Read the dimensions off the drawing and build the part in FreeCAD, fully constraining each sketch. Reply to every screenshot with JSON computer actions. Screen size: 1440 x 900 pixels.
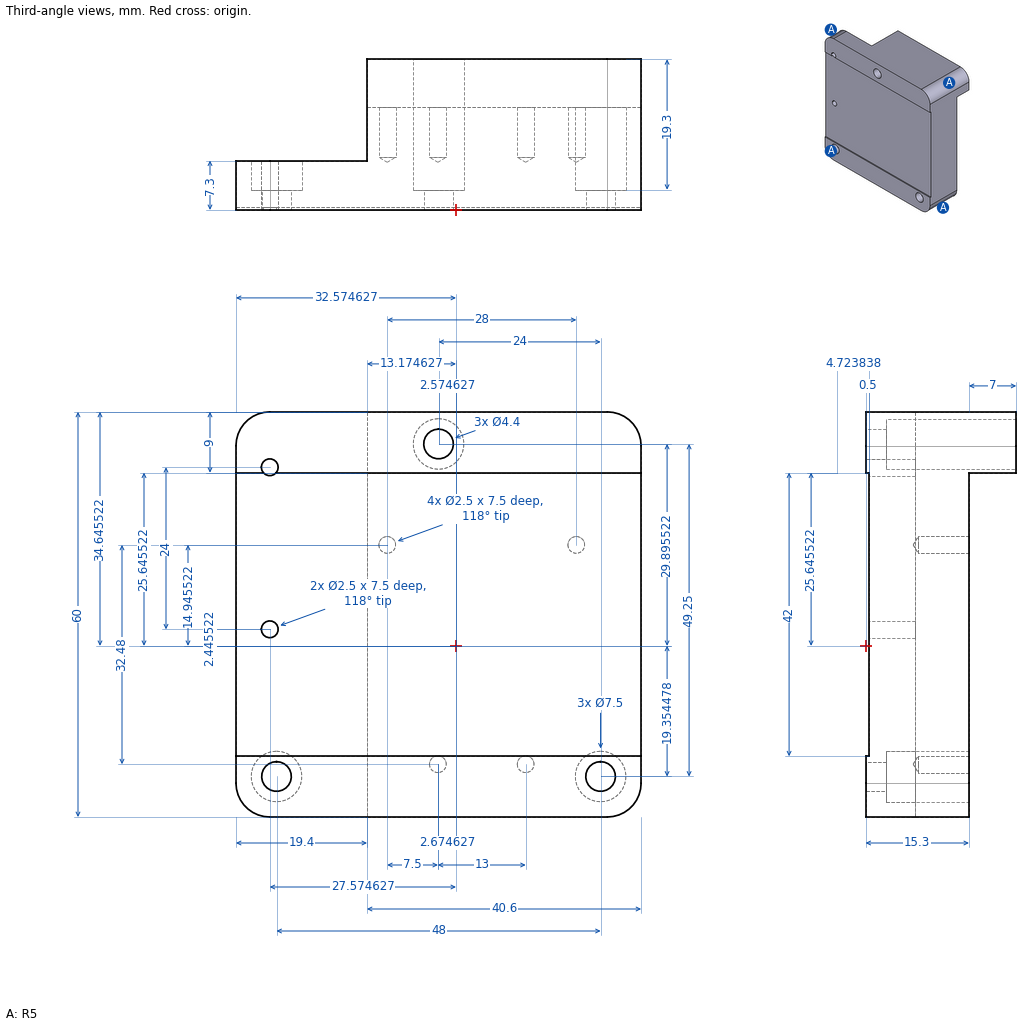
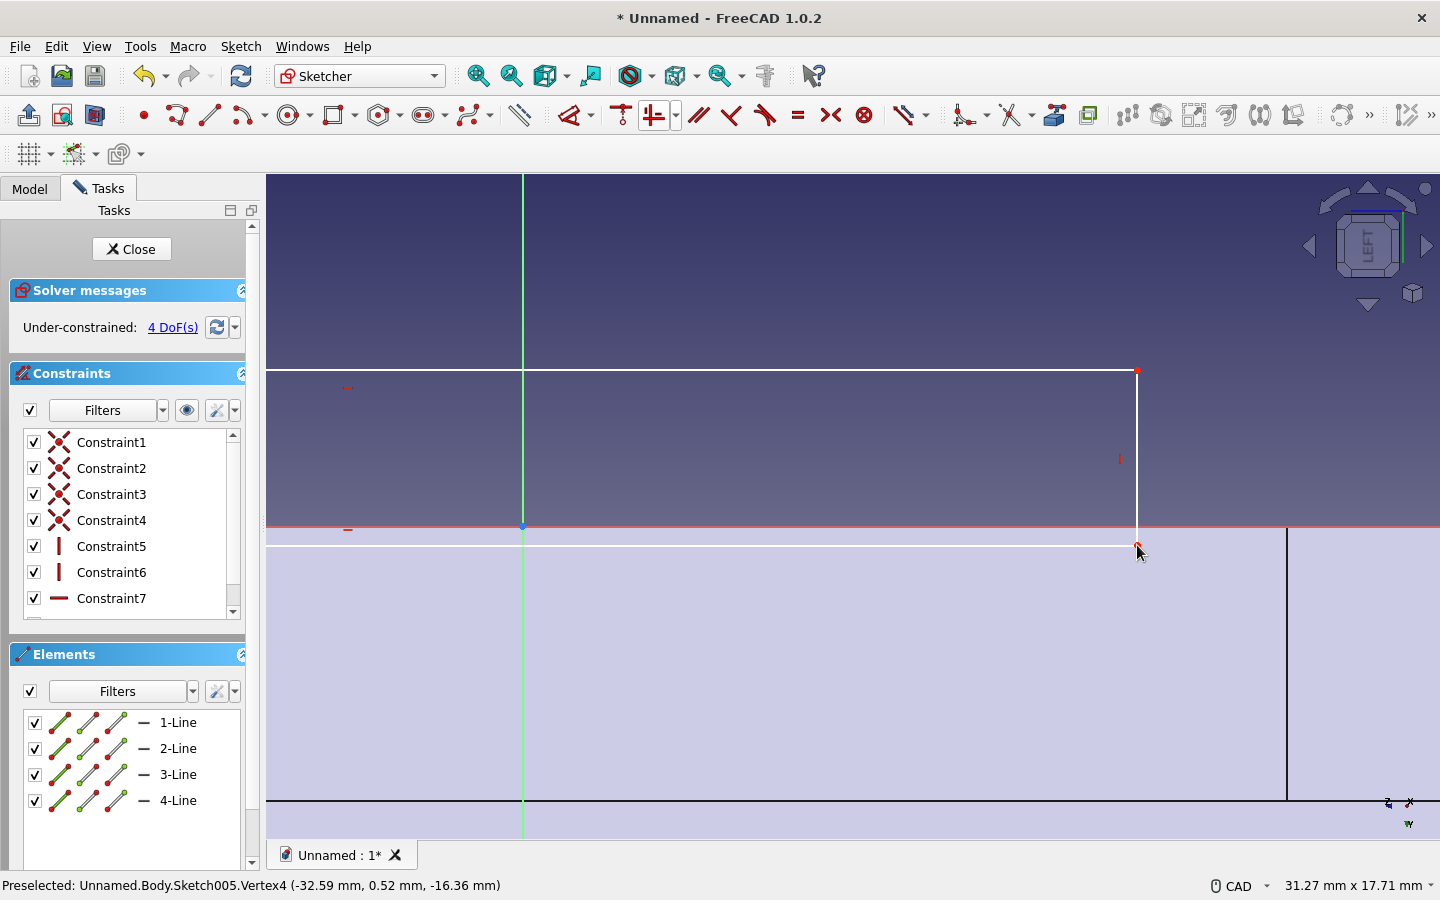
{"action": "key", "text": "d"}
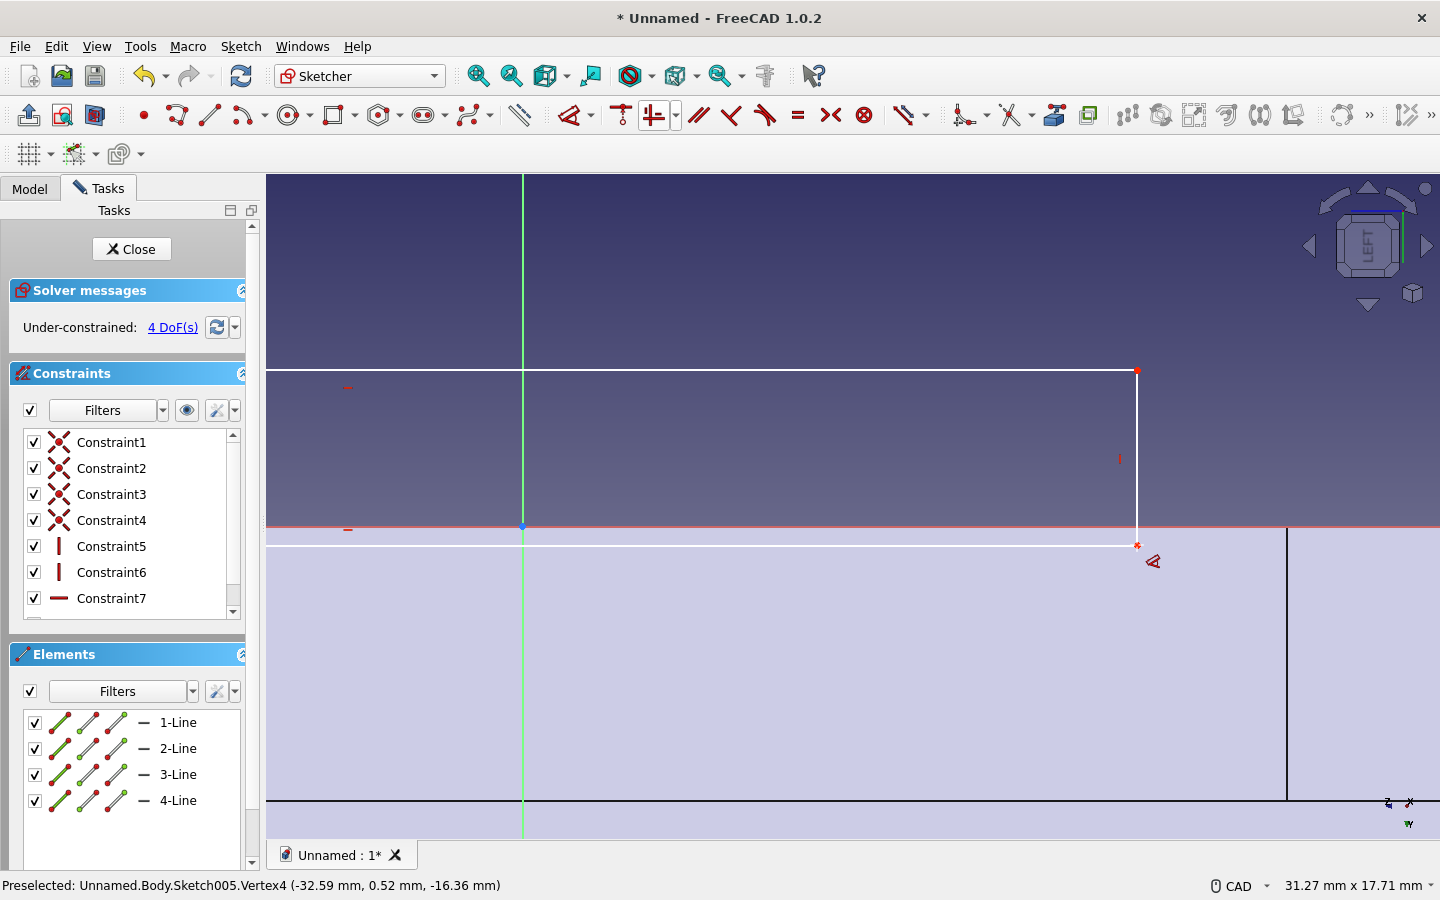
{"action": "left_click", "coordinate": [664, 546]}
{"action": "left_click", "coordinate": [715, 580]}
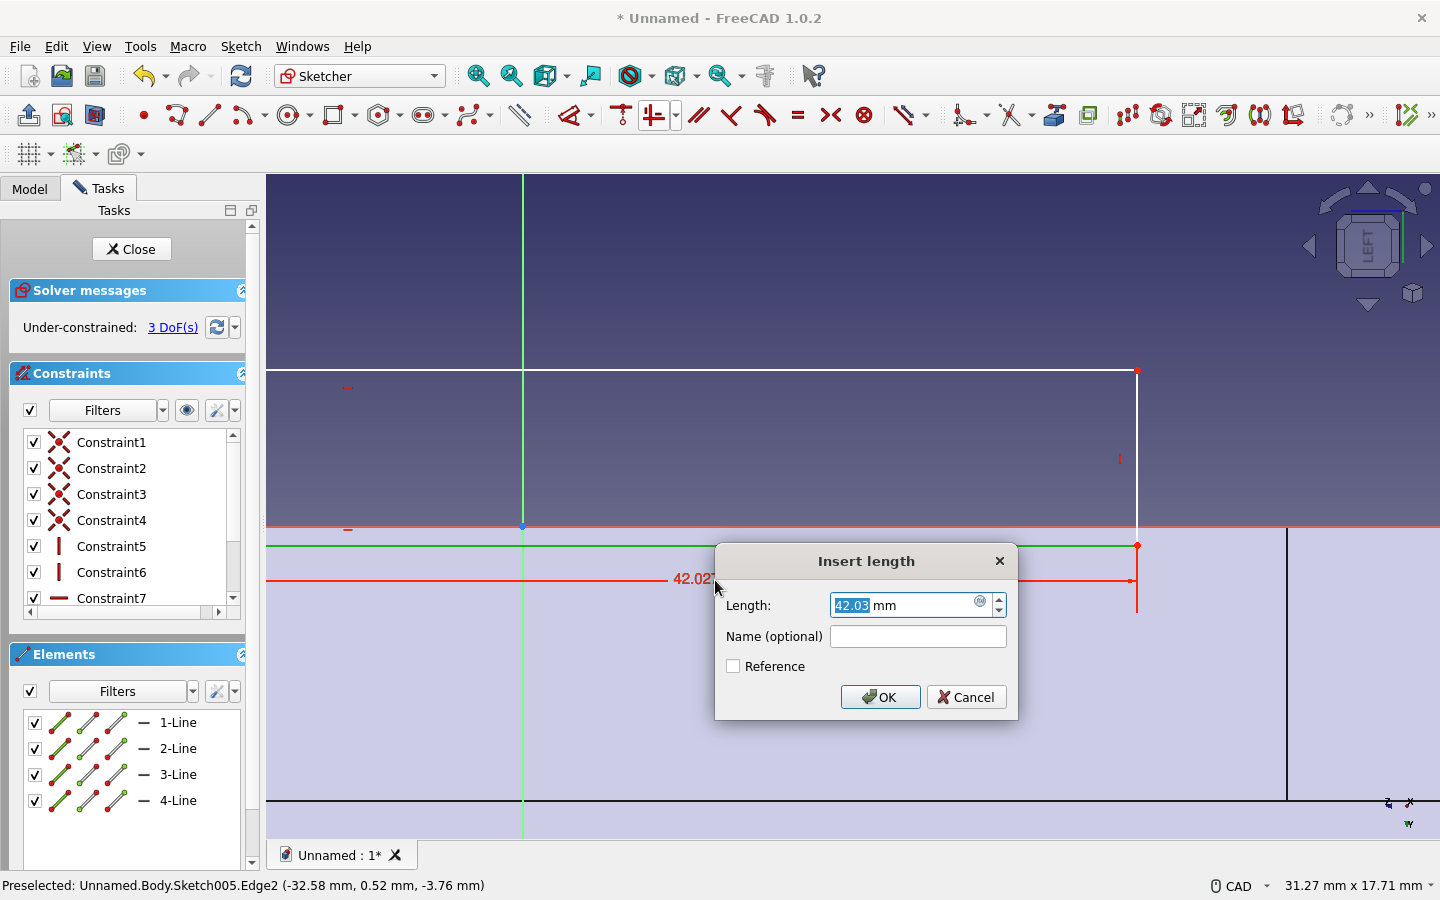
{"action": "type", "text": "42"}
{"action": "key", "text": "Return"}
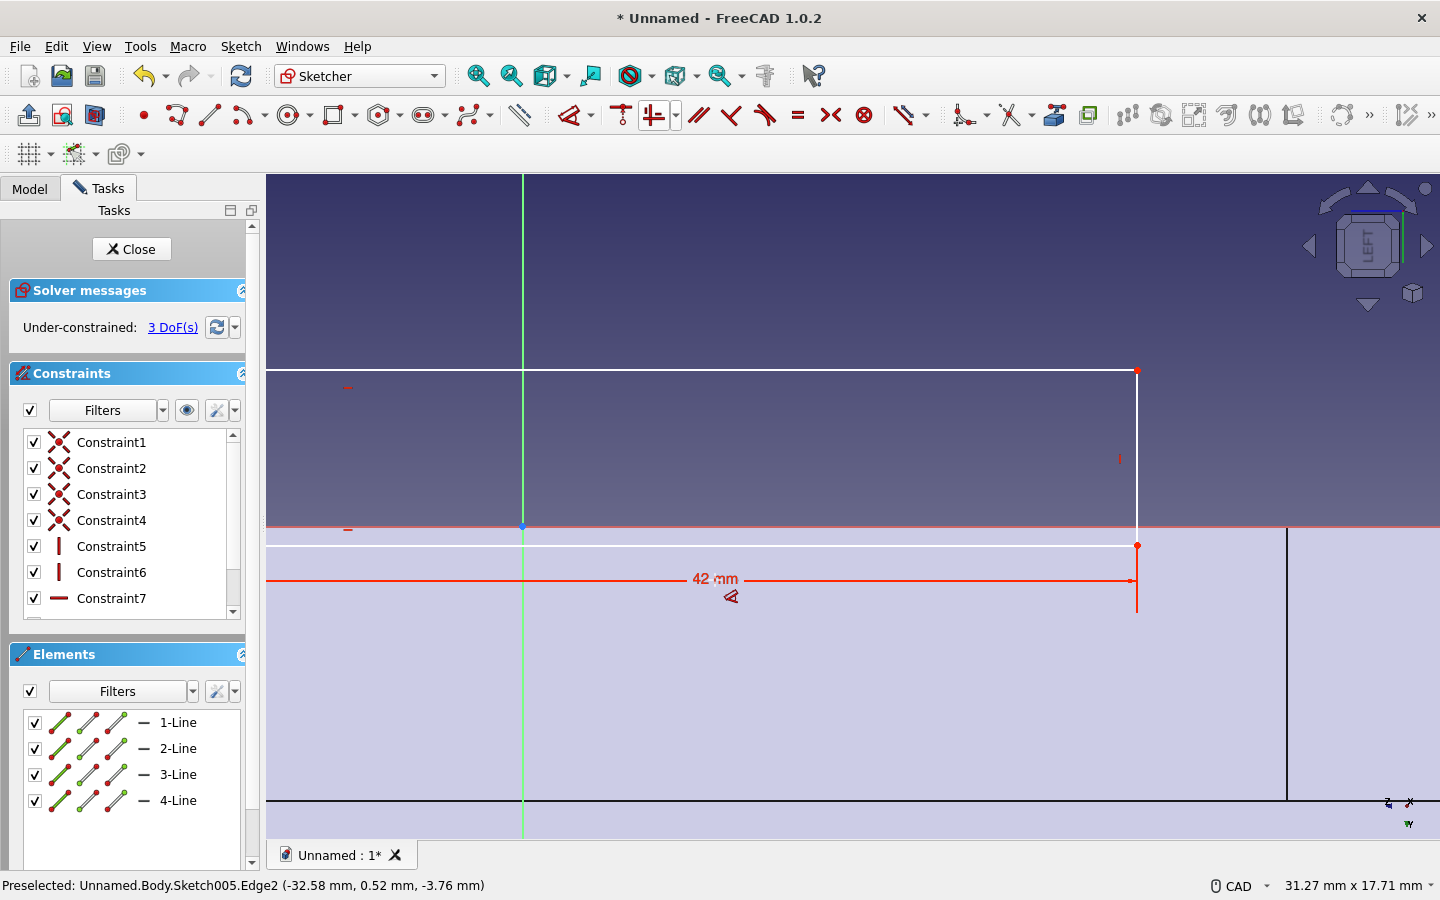
{"action": "scroll", "coordinate": [1140, 547], "scroll_direction": "down", "scroll_amount": 4}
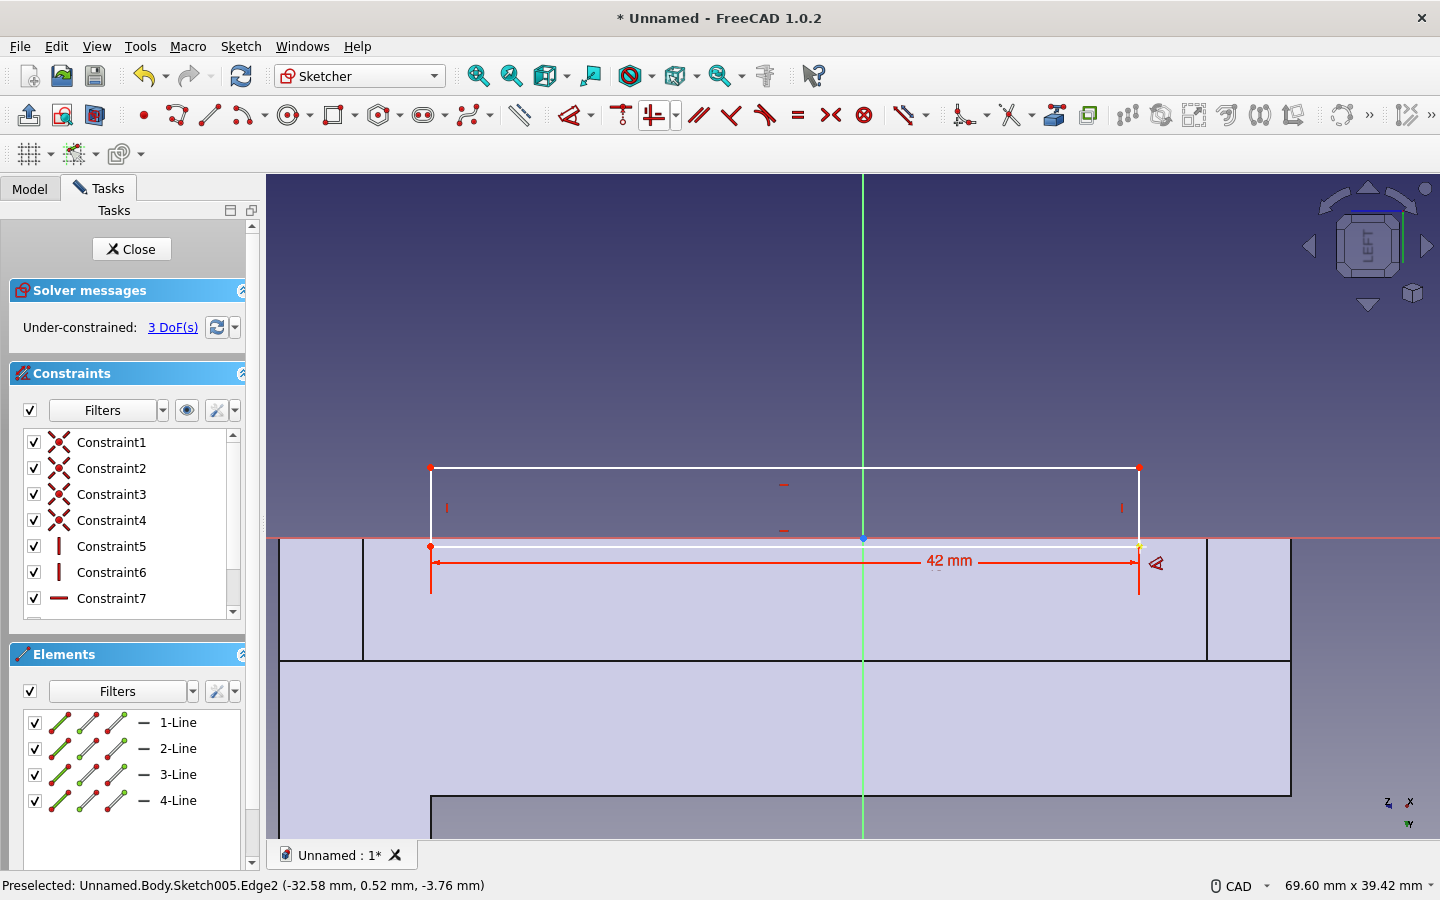
{"action": "scroll", "coordinate": [431, 547], "scroll_direction": "up", "scroll_amount": 8}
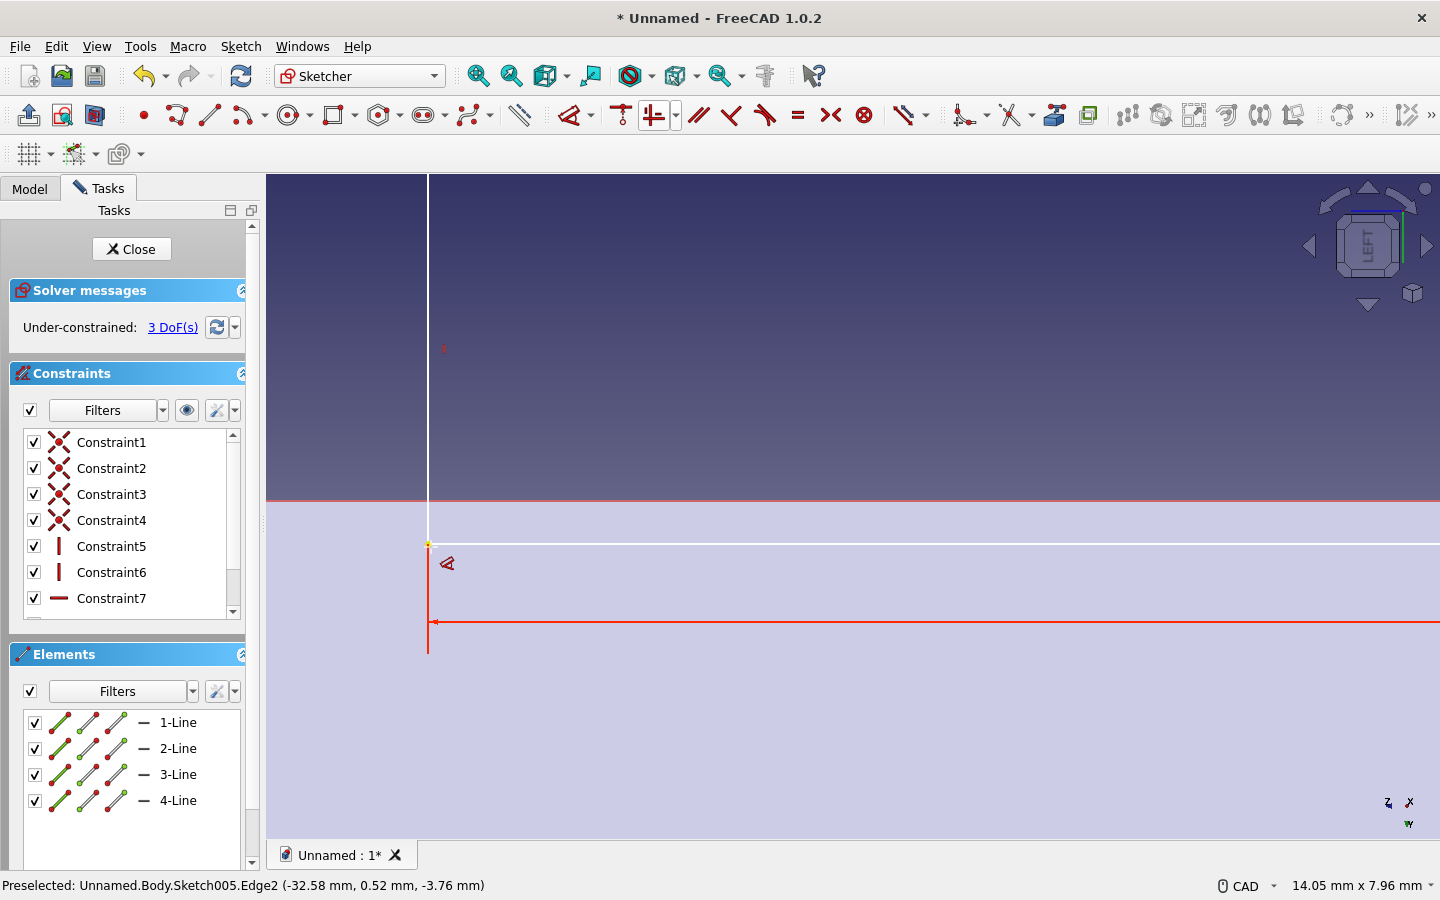
{"action": "left_click", "coordinate": [428, 544]}
{"action": "left_click", "coordinate": [394, 522]}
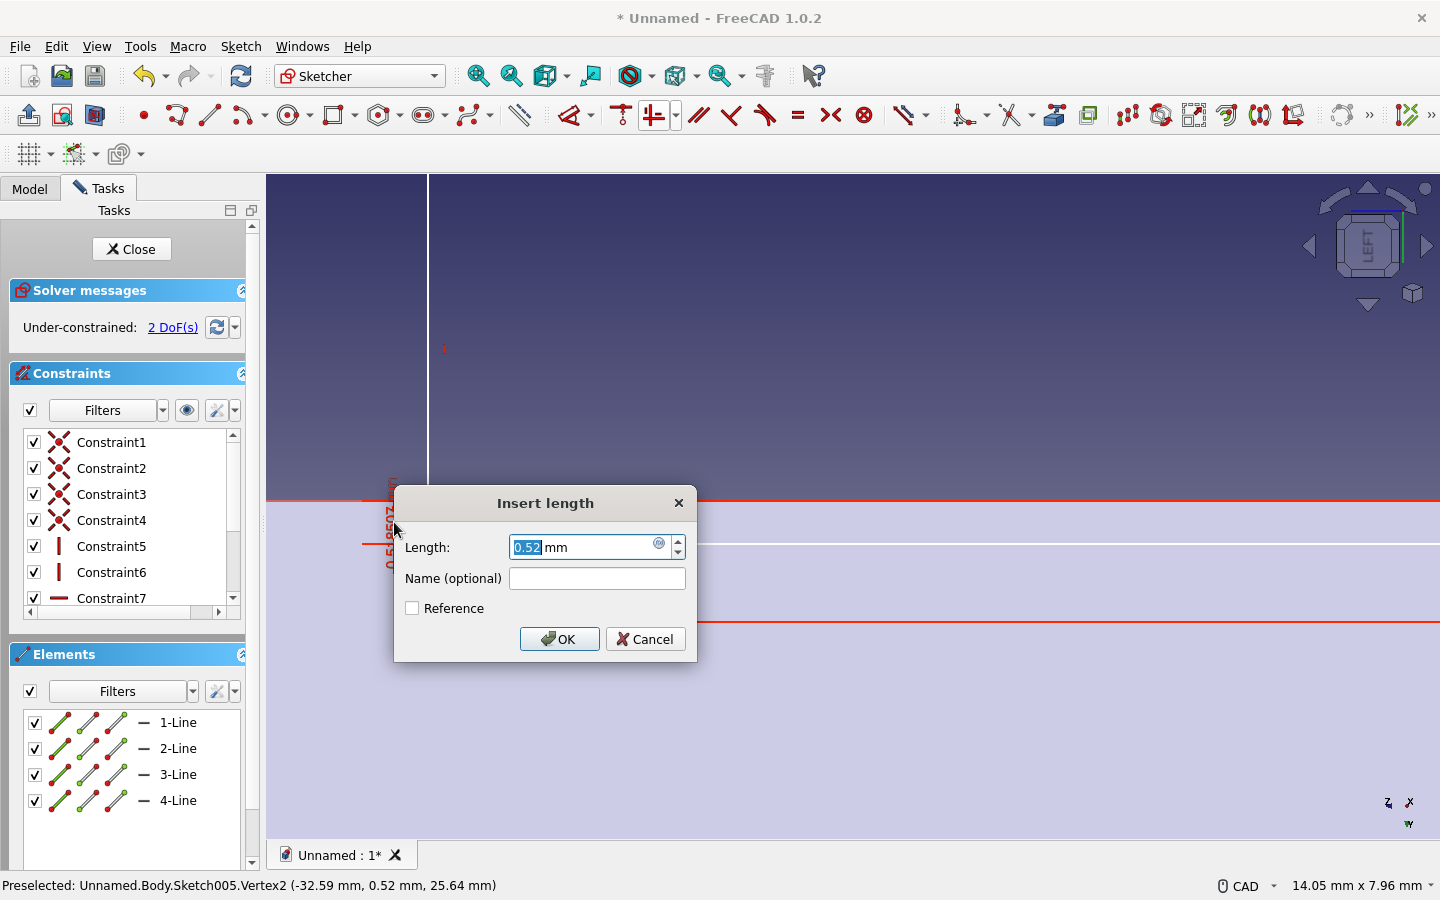
{"action": "type", "text": "0.5"}
{"action": "key", "text": "Return"}